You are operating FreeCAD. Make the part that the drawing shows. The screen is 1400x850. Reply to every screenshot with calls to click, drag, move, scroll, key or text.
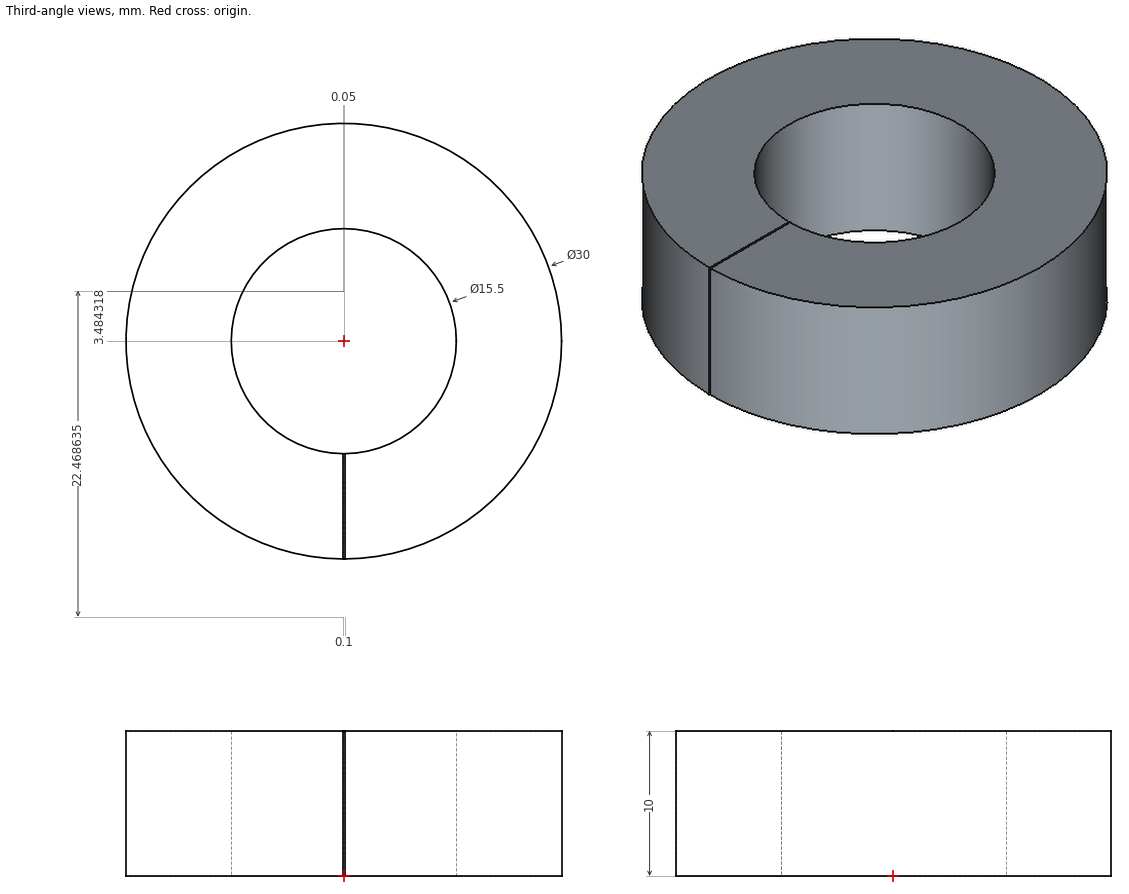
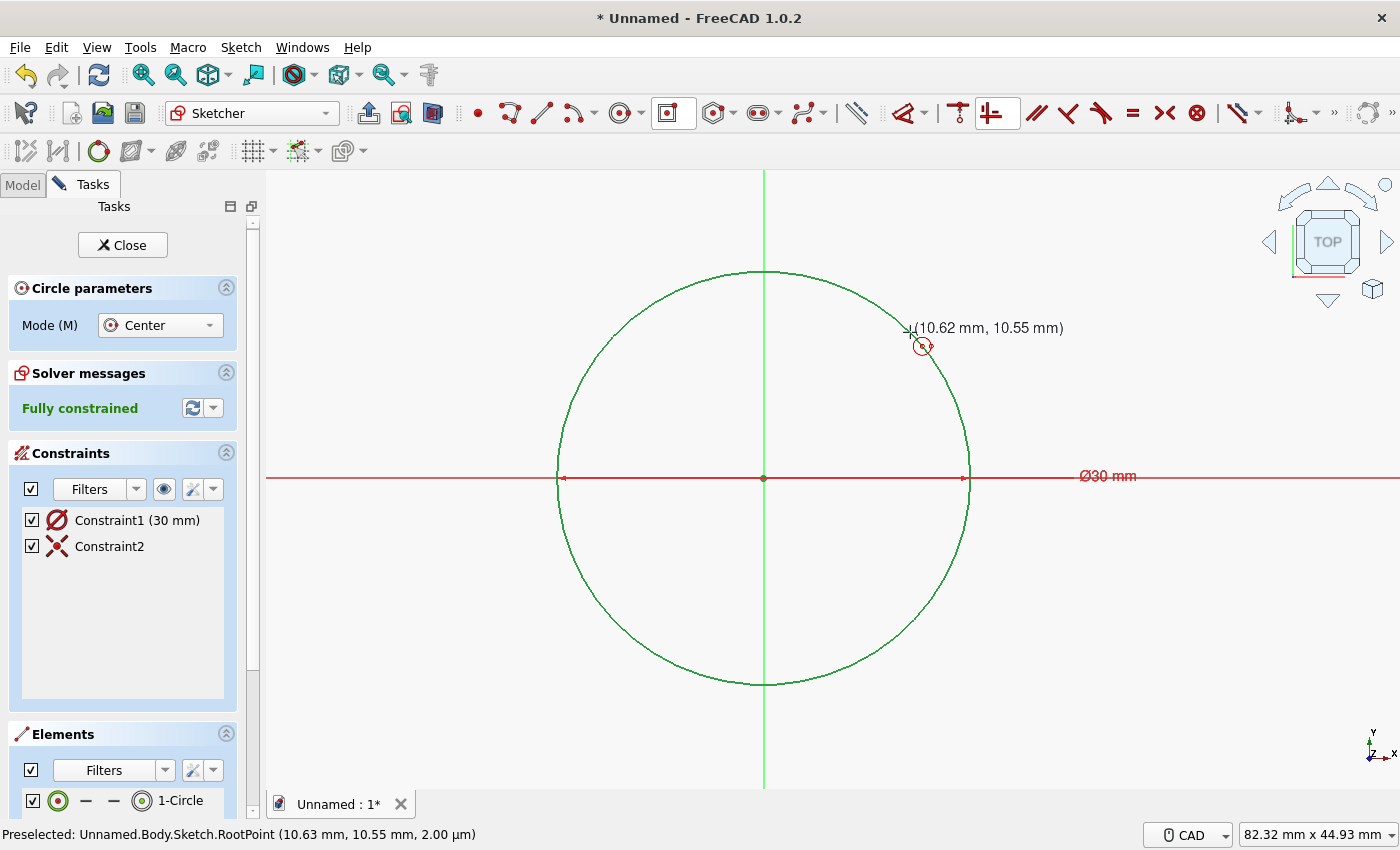
click(764, 478)
move(839, 403)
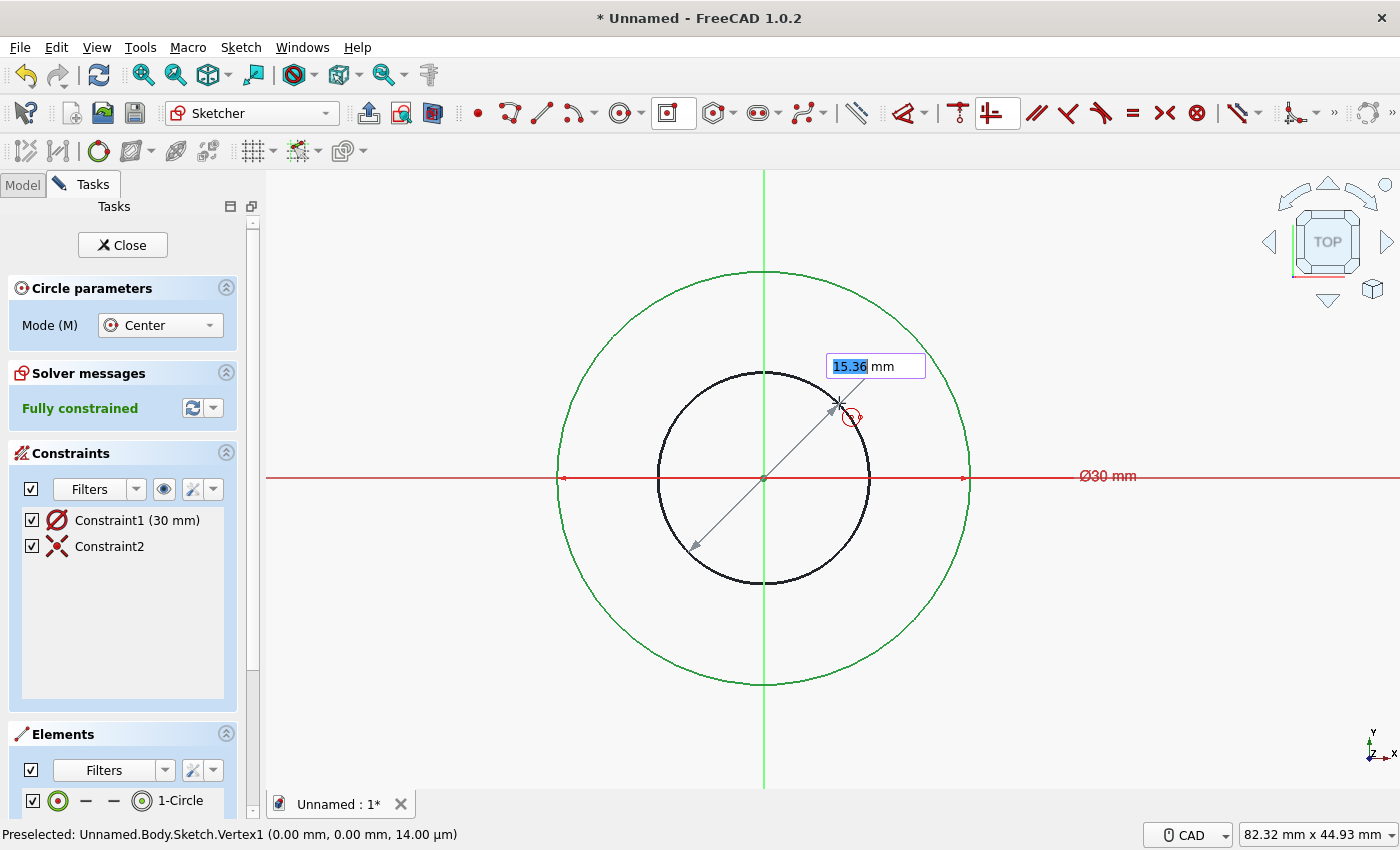
text(15.5)
key(Return)
key(Escape)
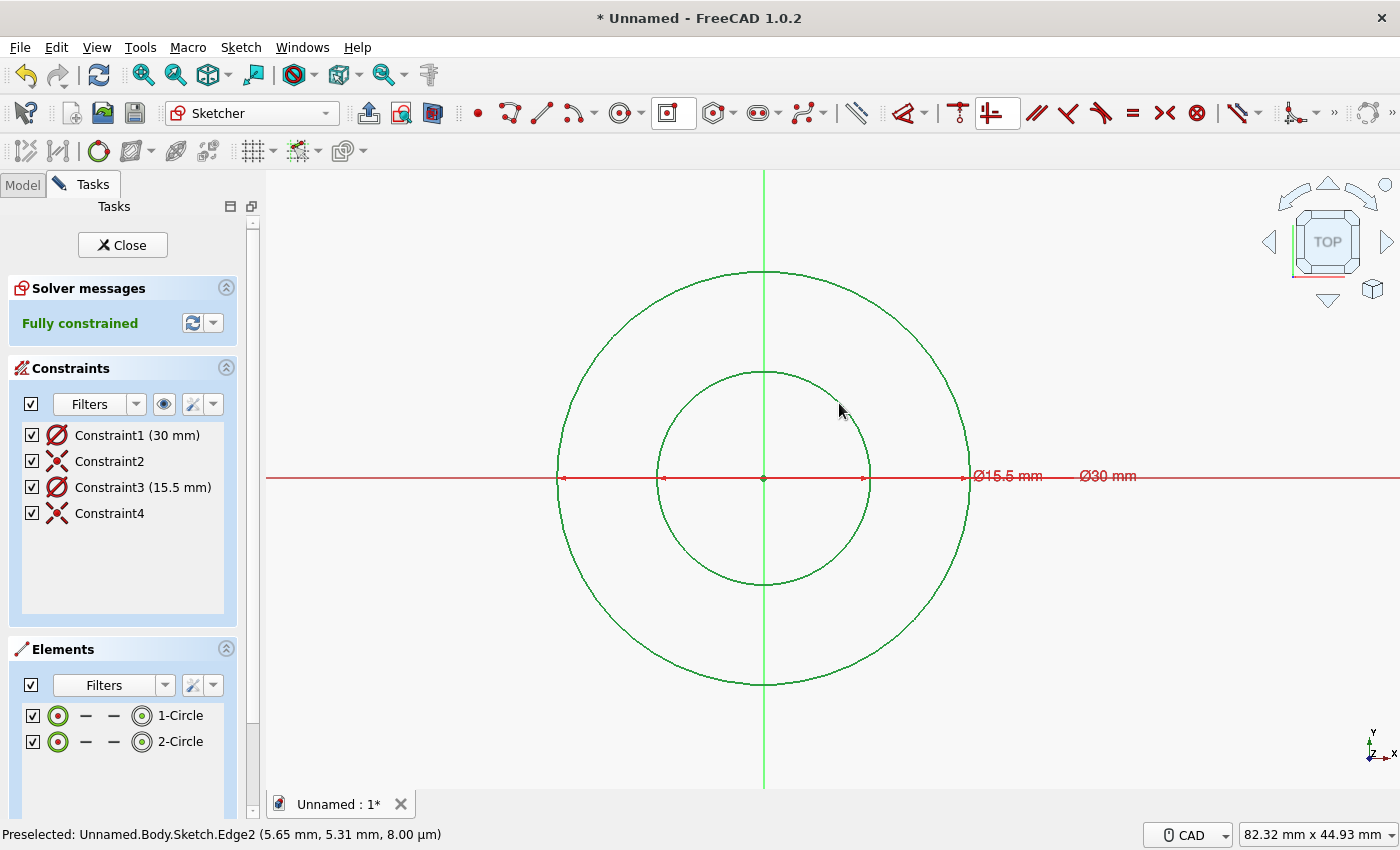
click(123, 245)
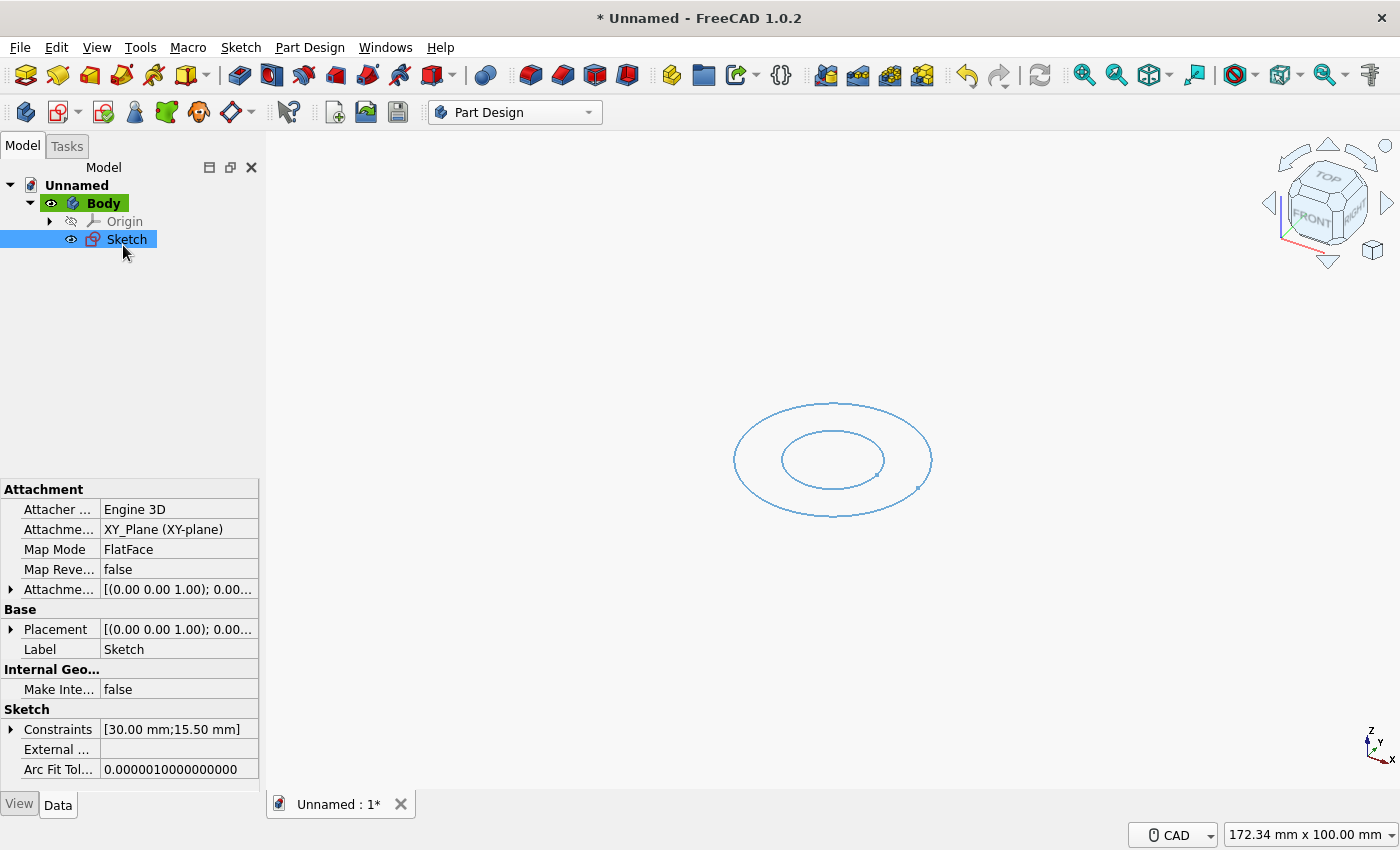
click(26, 76)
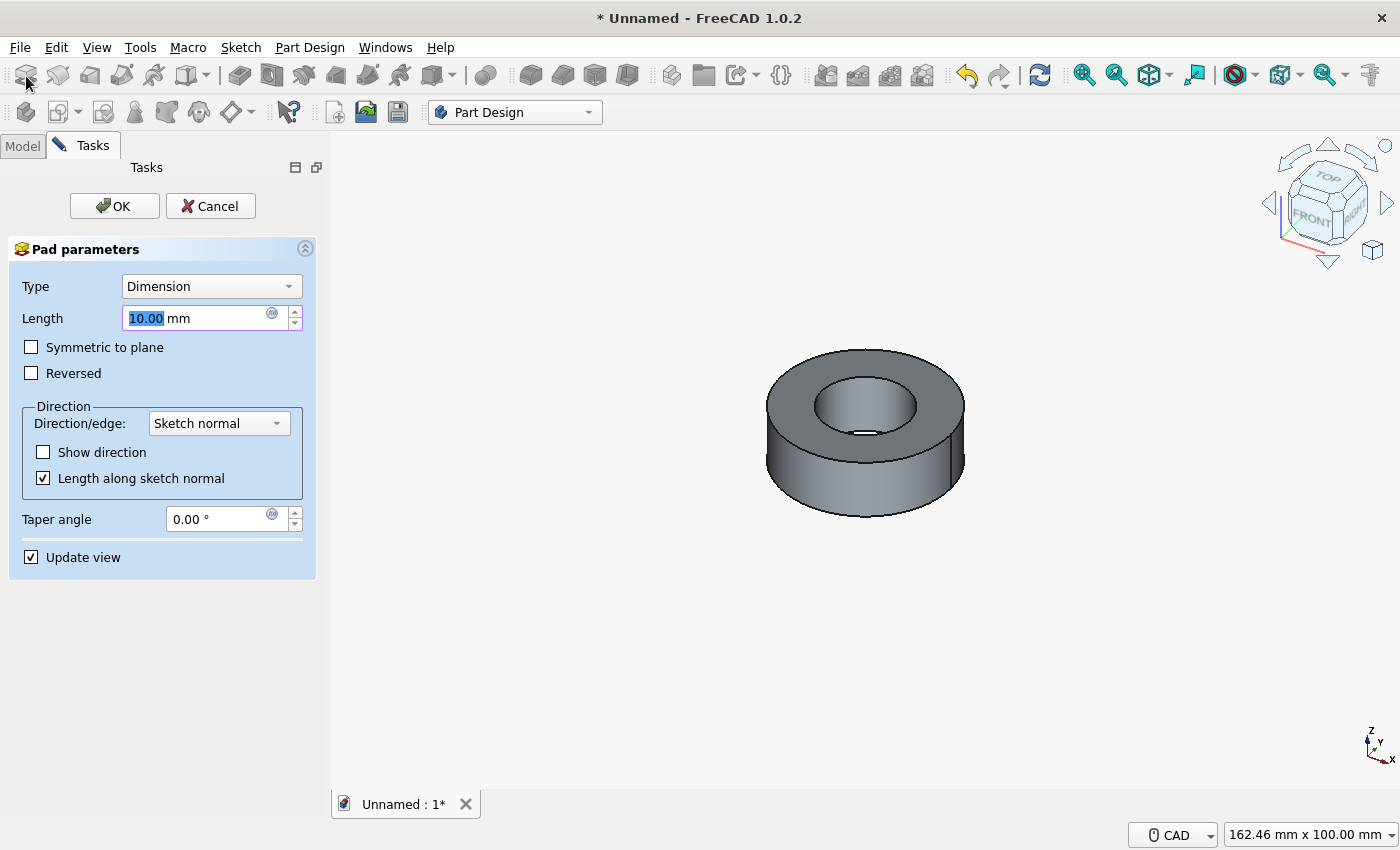
text(10)
key(Tab)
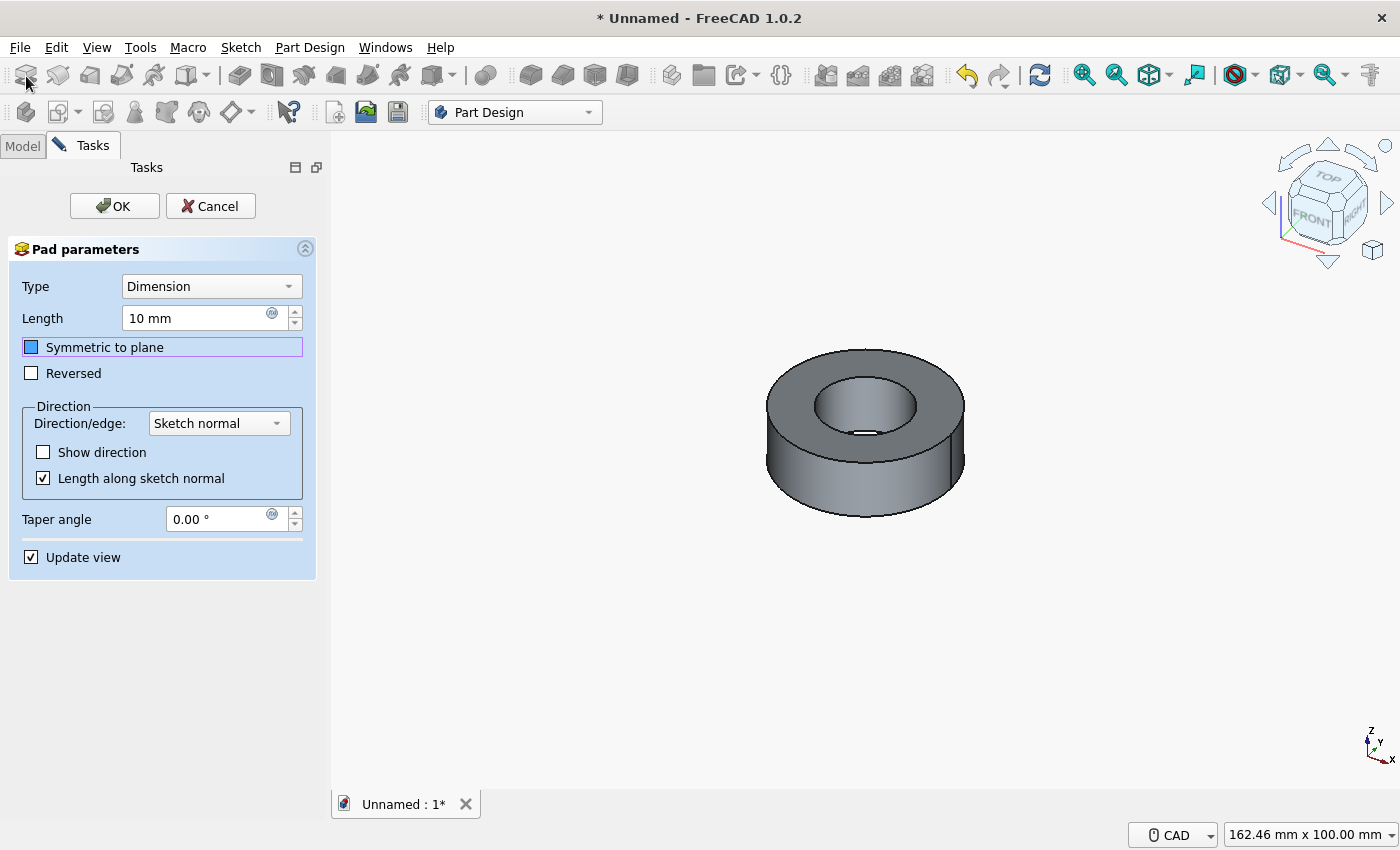
click(115, 206)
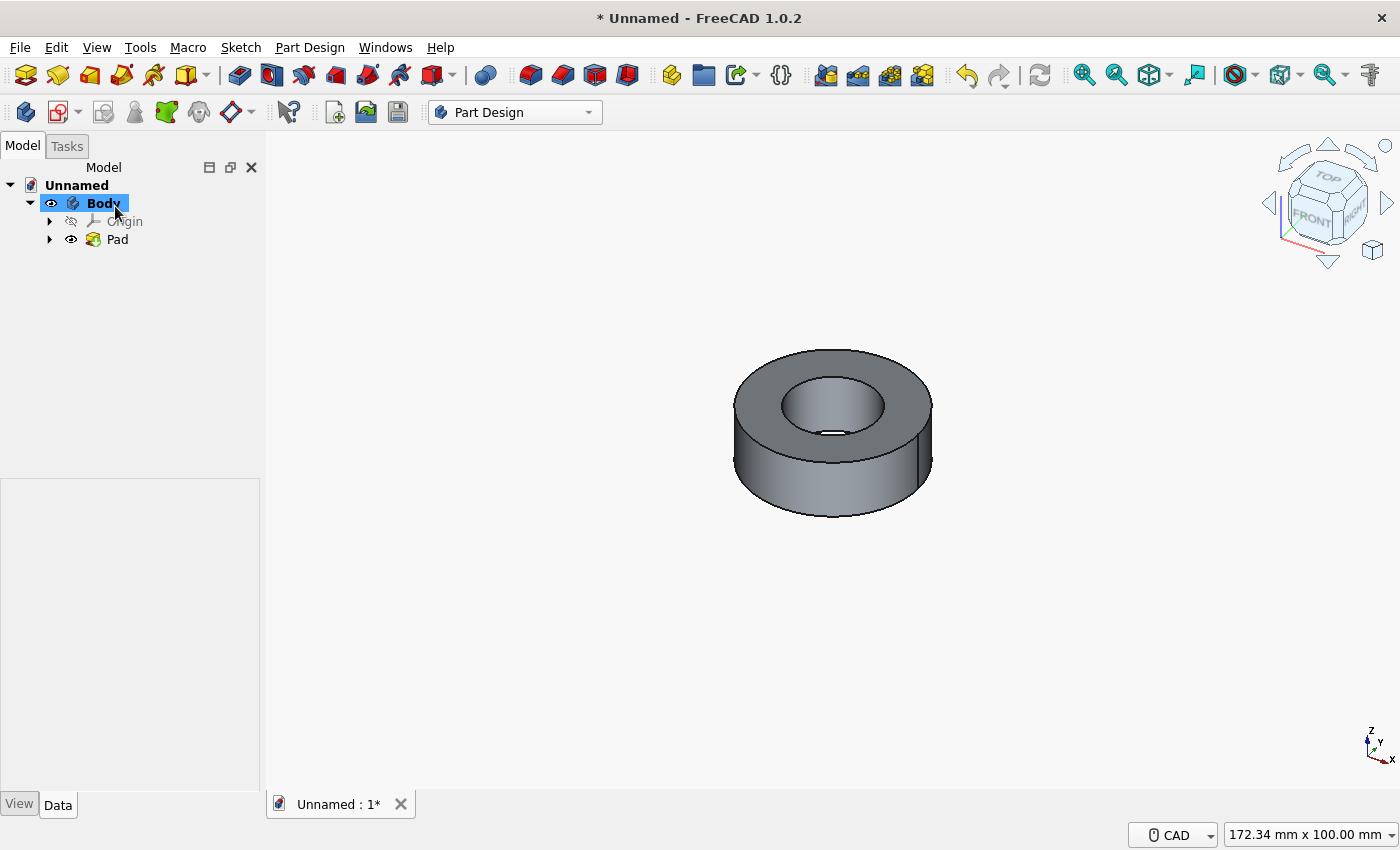
click(1086, 76)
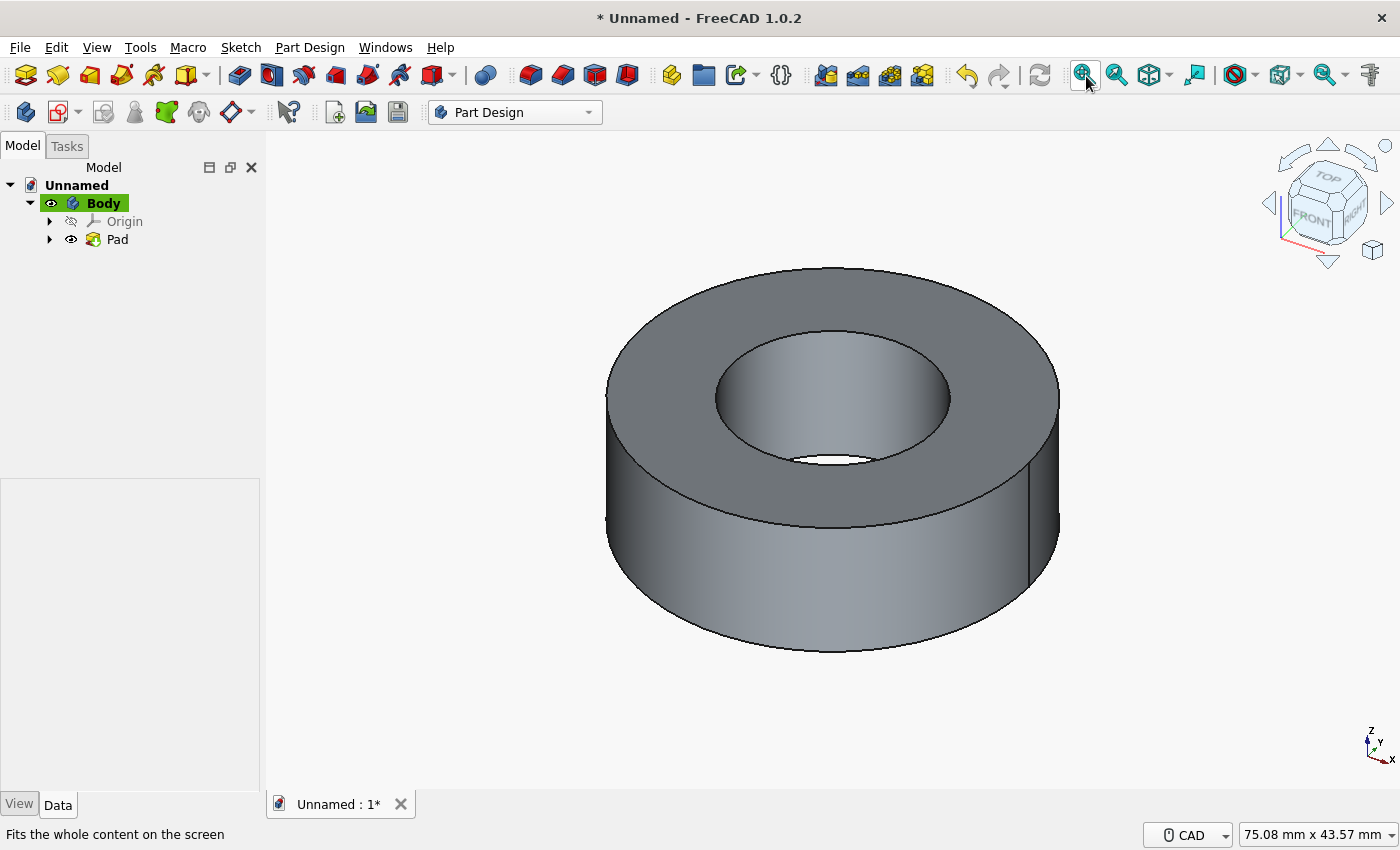
click(656, 424)